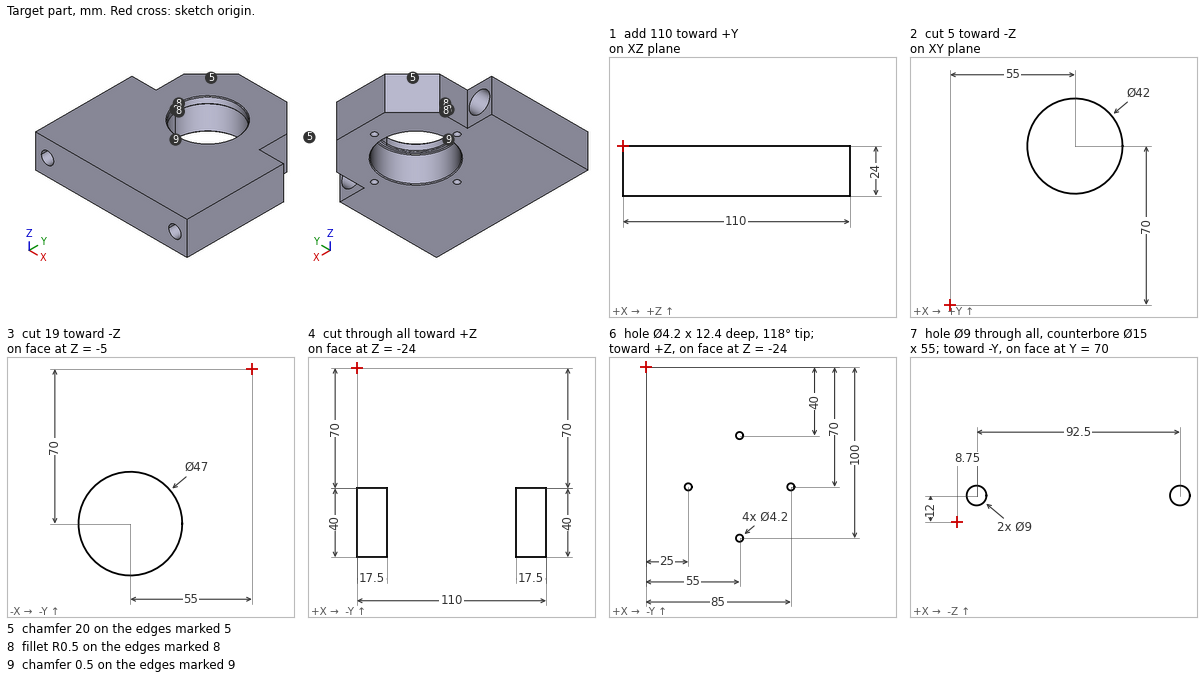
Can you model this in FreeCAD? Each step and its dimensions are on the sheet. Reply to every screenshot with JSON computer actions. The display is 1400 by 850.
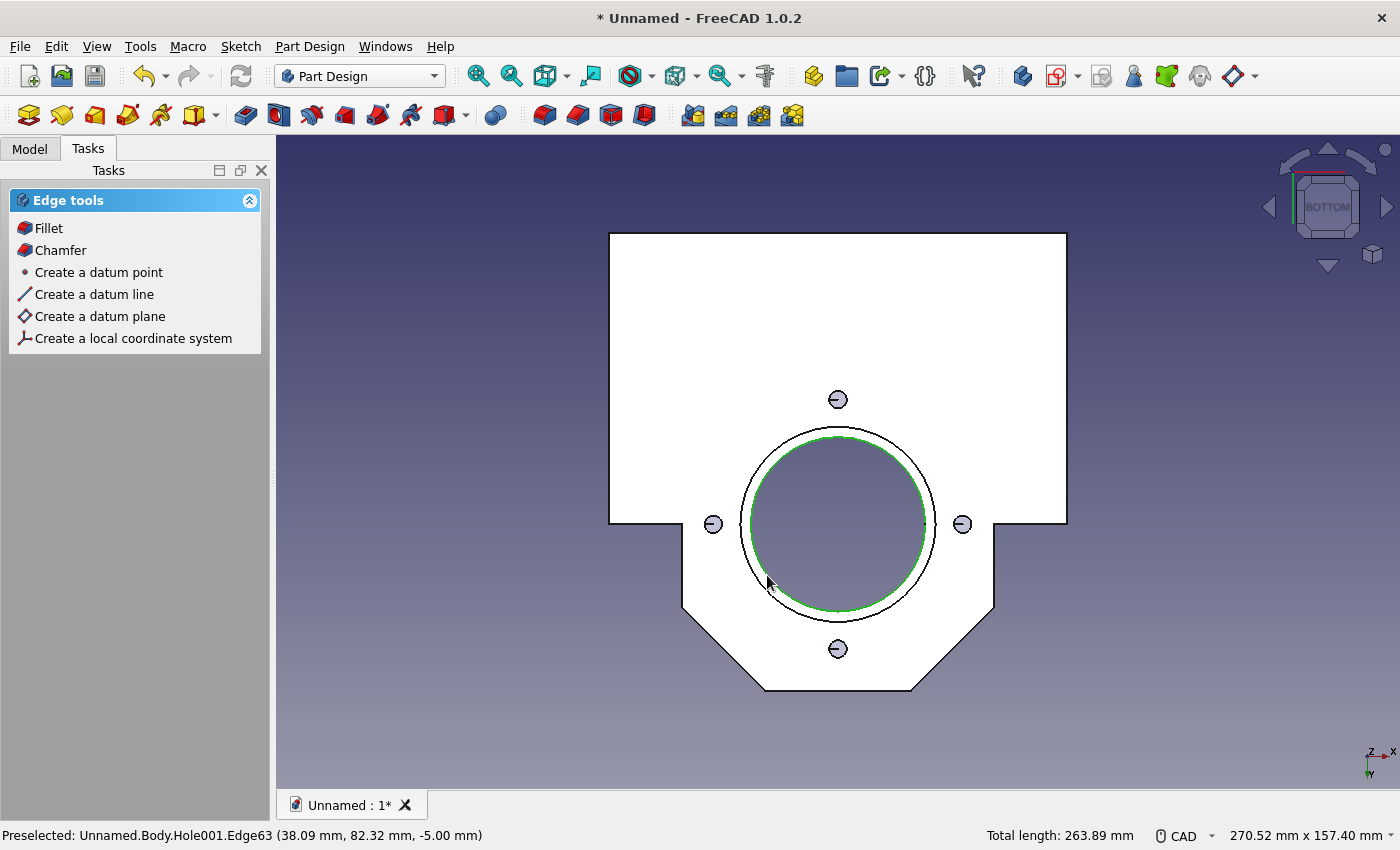
{"action": "key", "text": "4"}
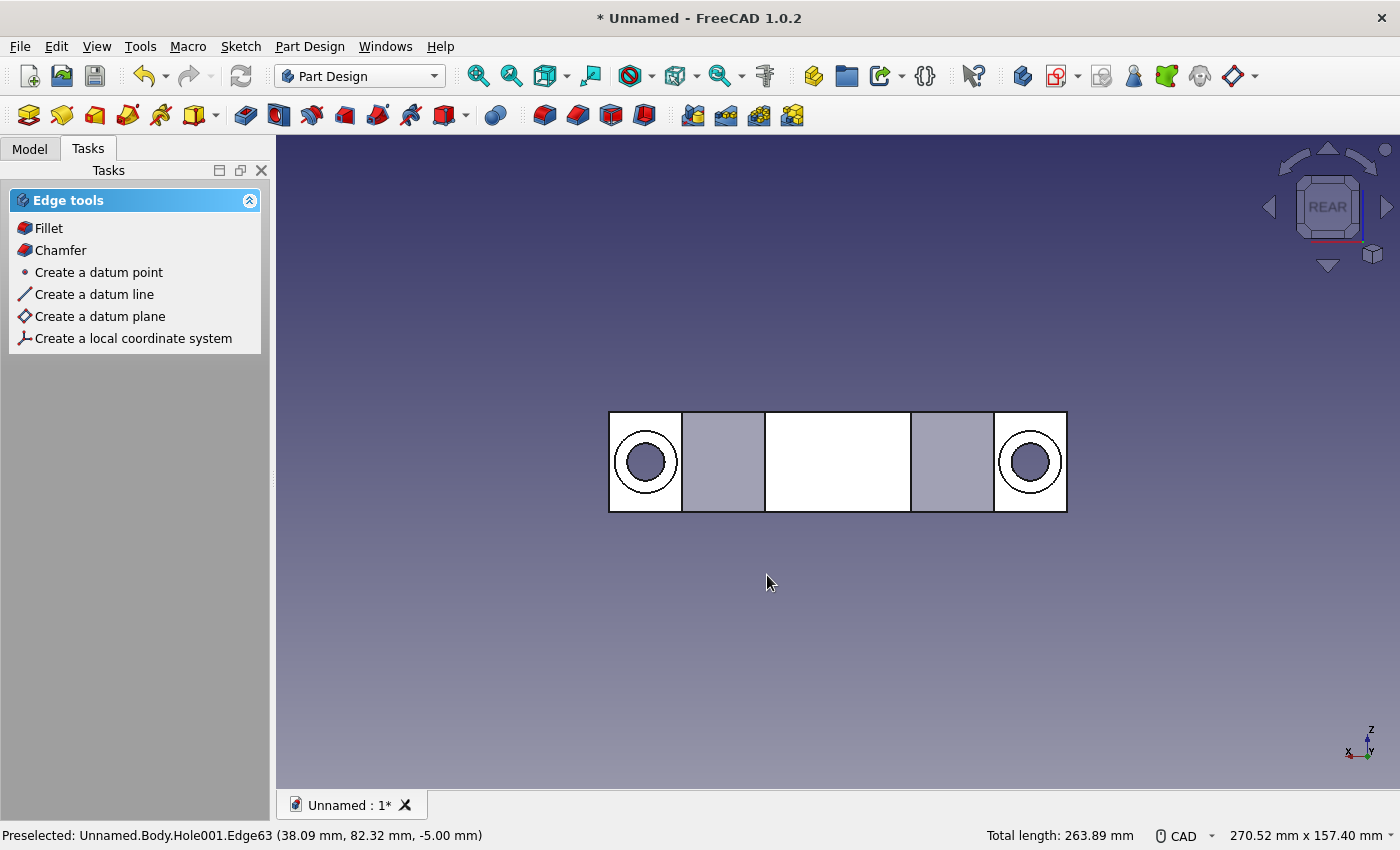
{"action": "left_click", "coordinate": [479, 76]}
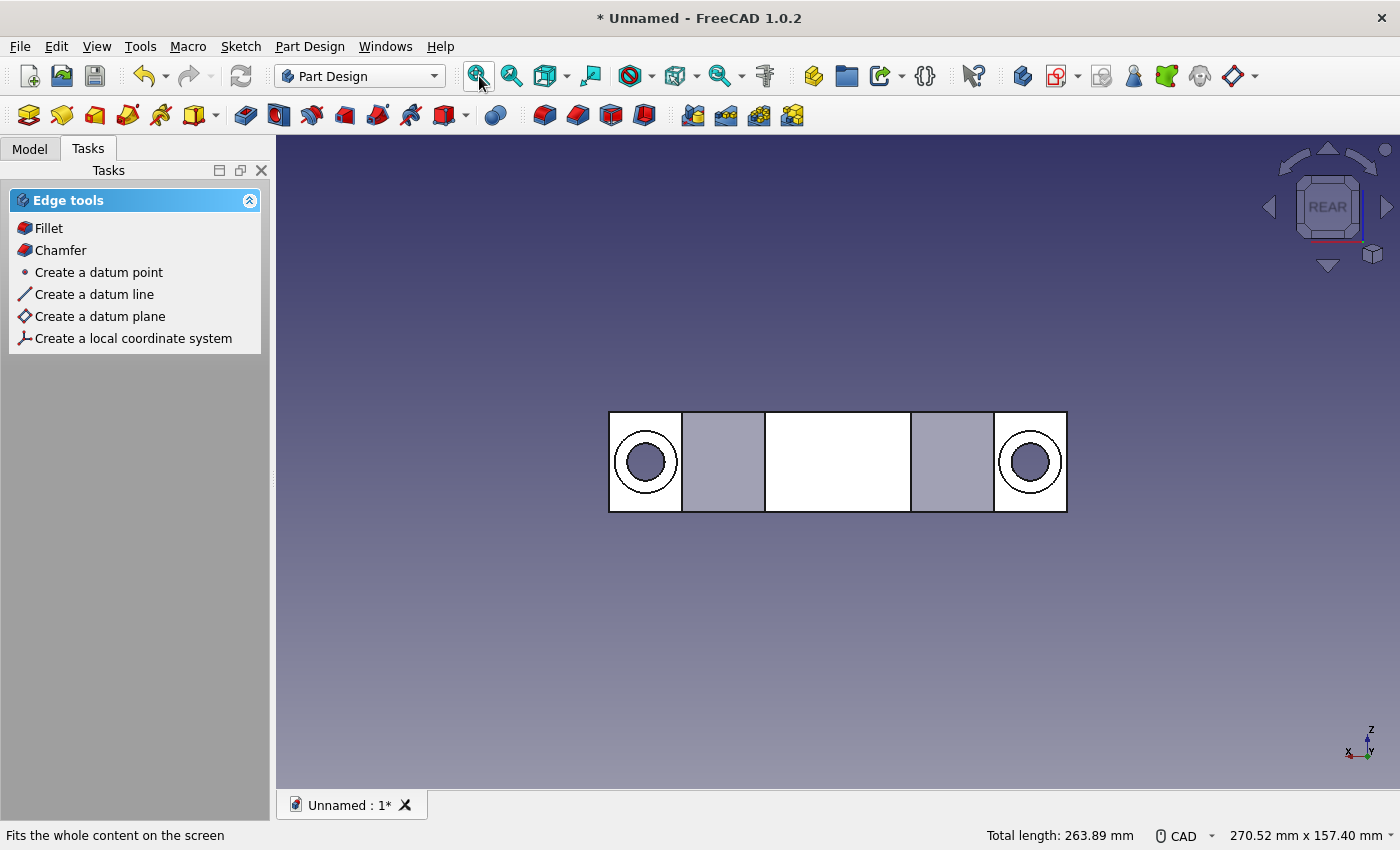
{"action": "key", "text": "6"}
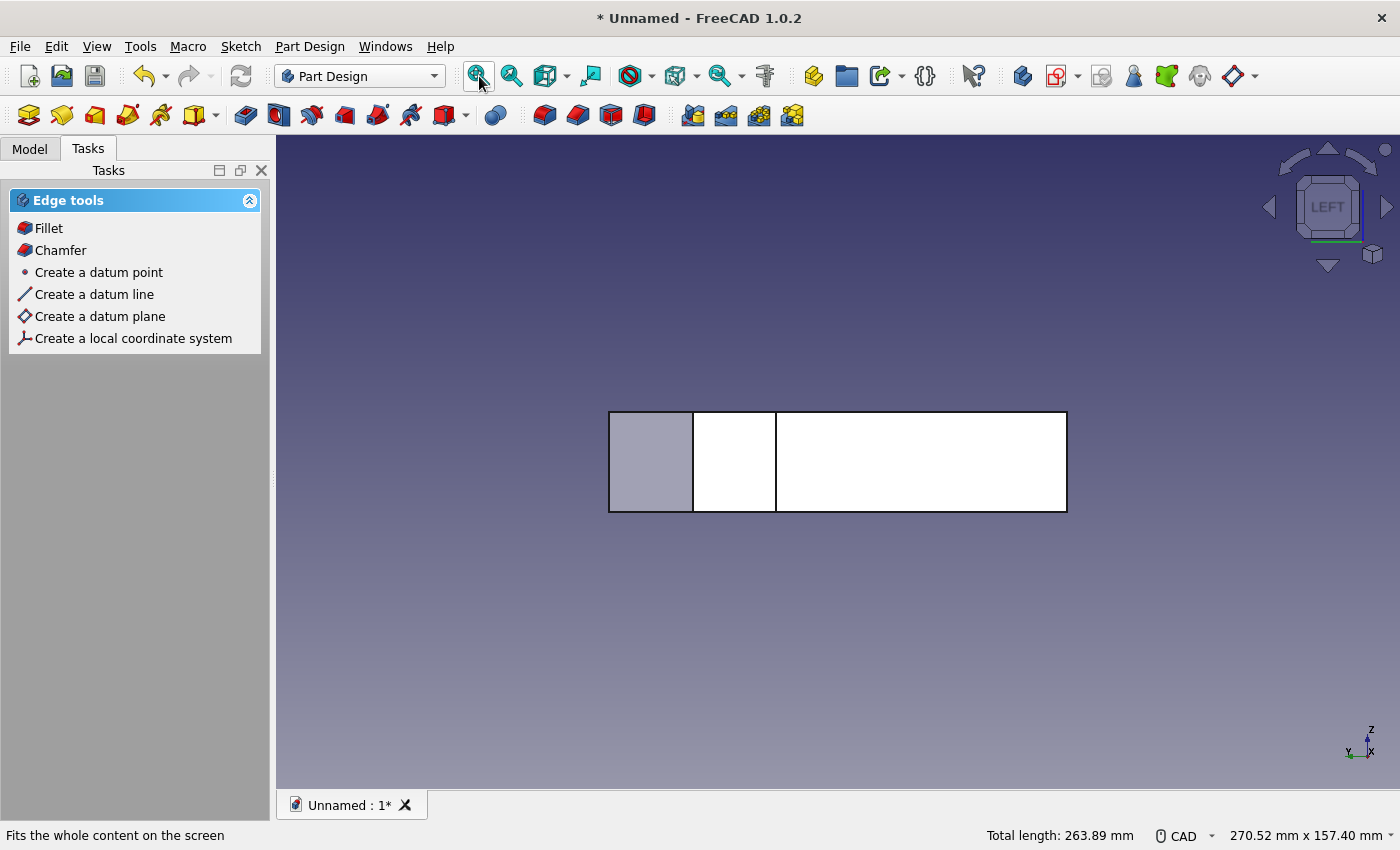
{"action": "key", "text": "v f"}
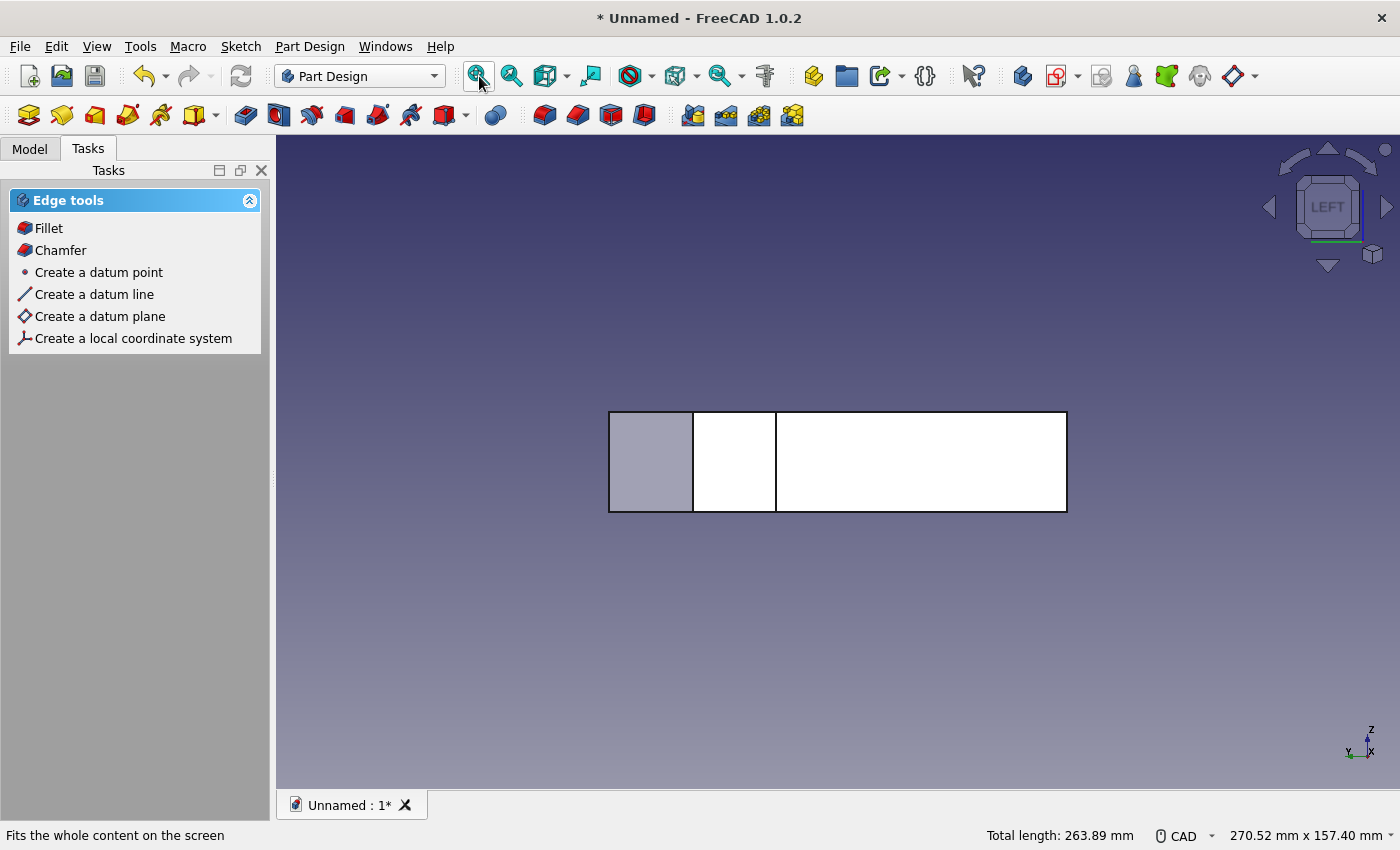
{"action": "key", "text": "v 3"}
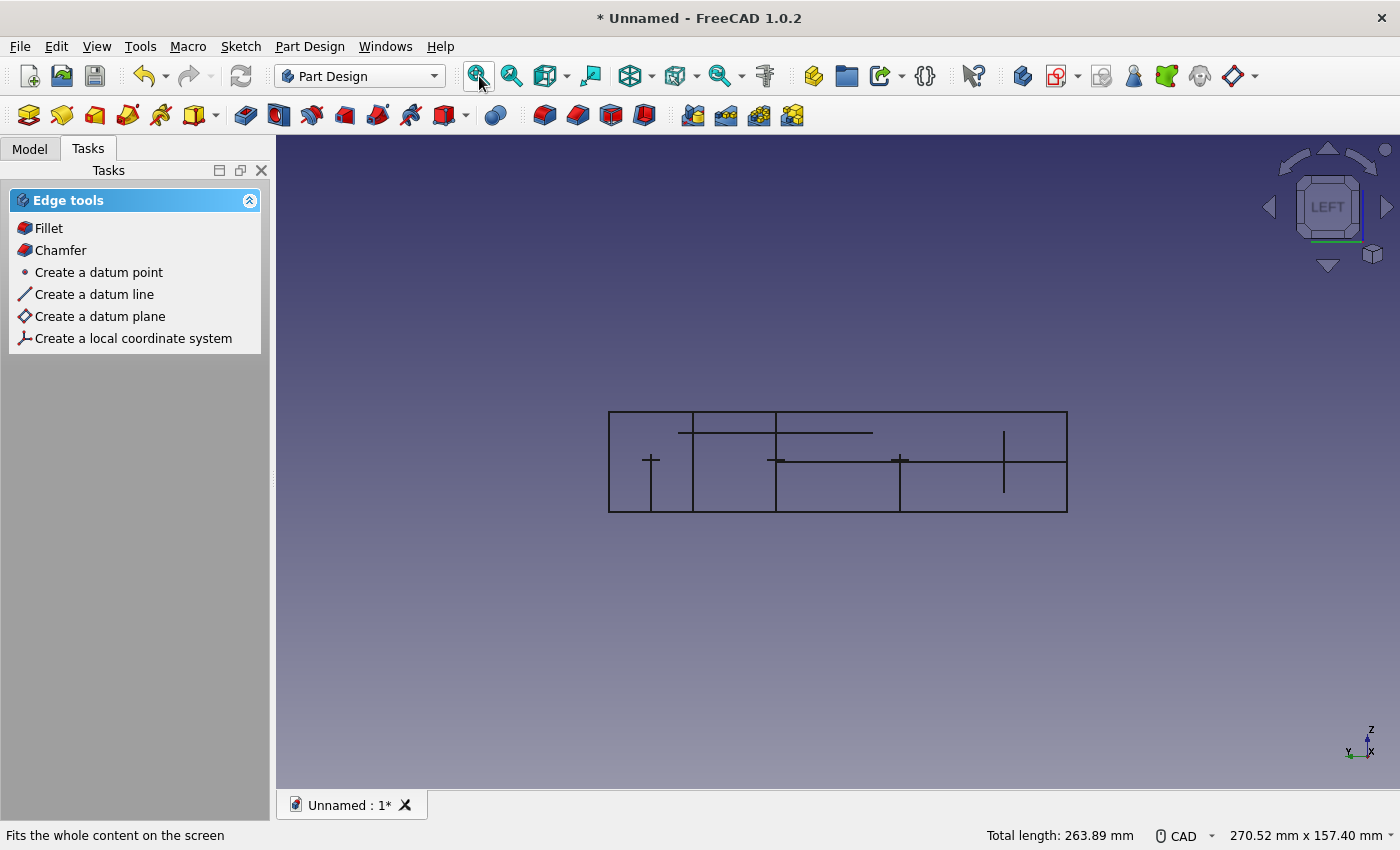
{"action": "key", "text": "0"}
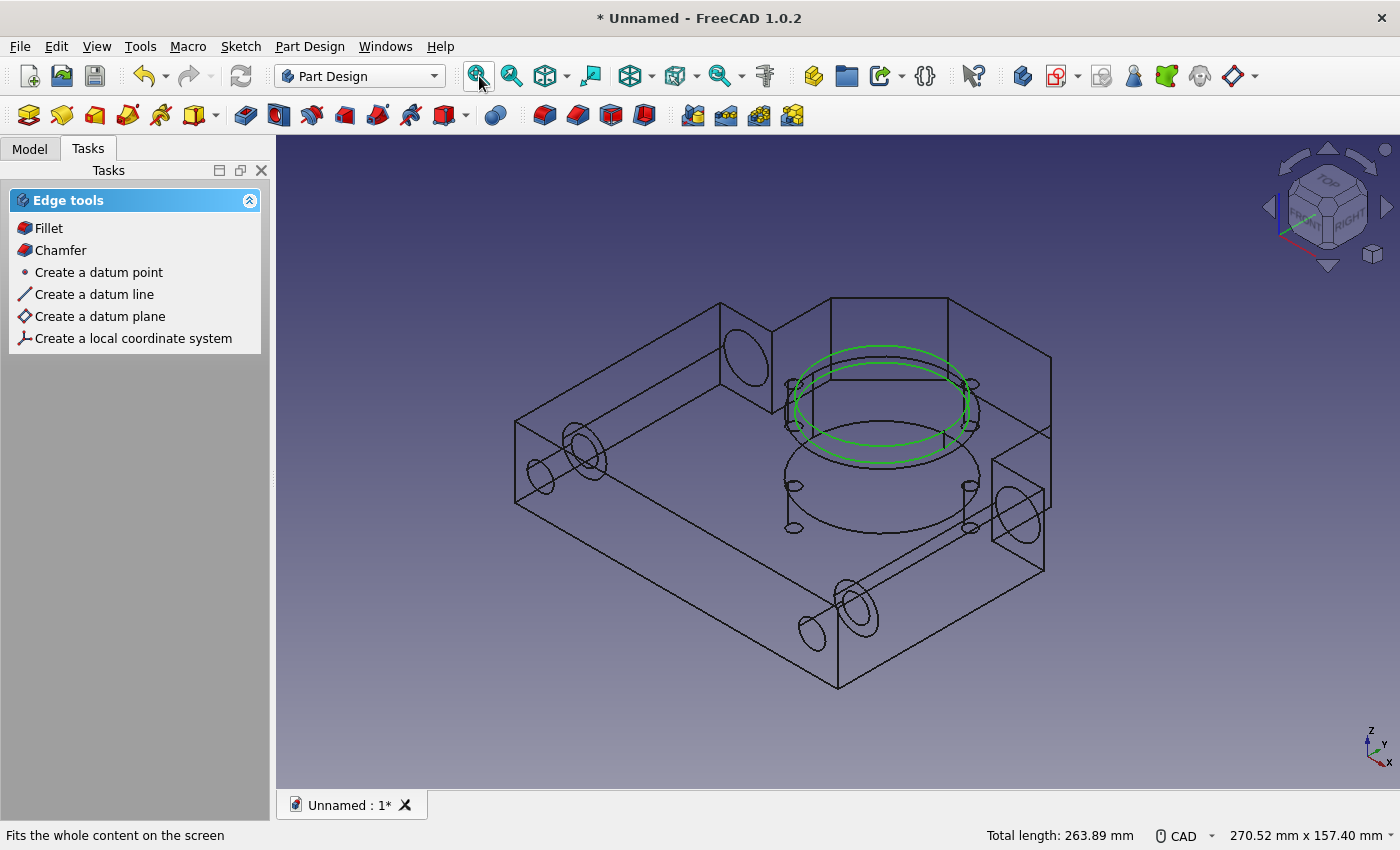
{"action": "left_click", "coordinate": [951, 452], "text": "ctrl"}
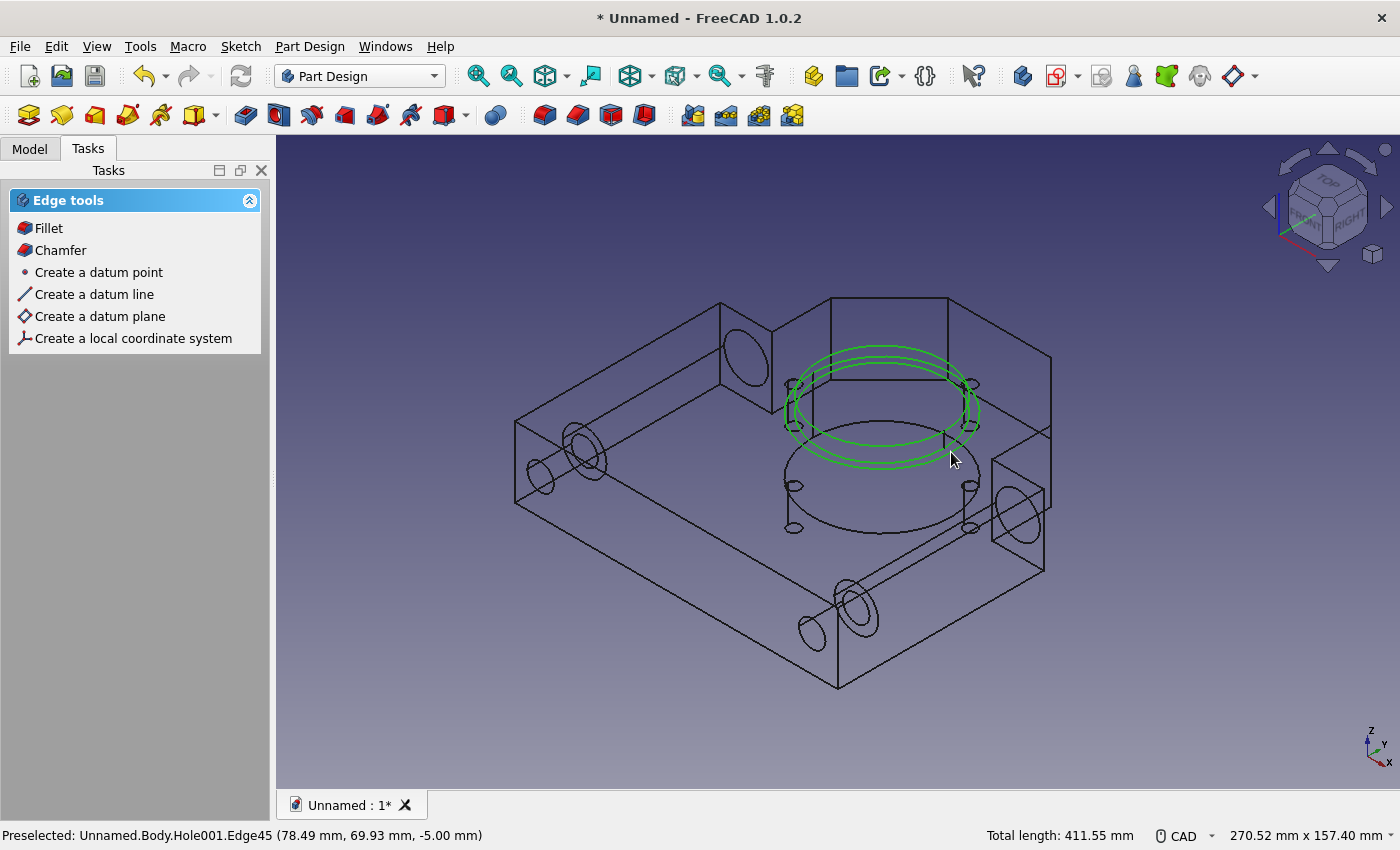
{"action": "key", "text": "v 1"}